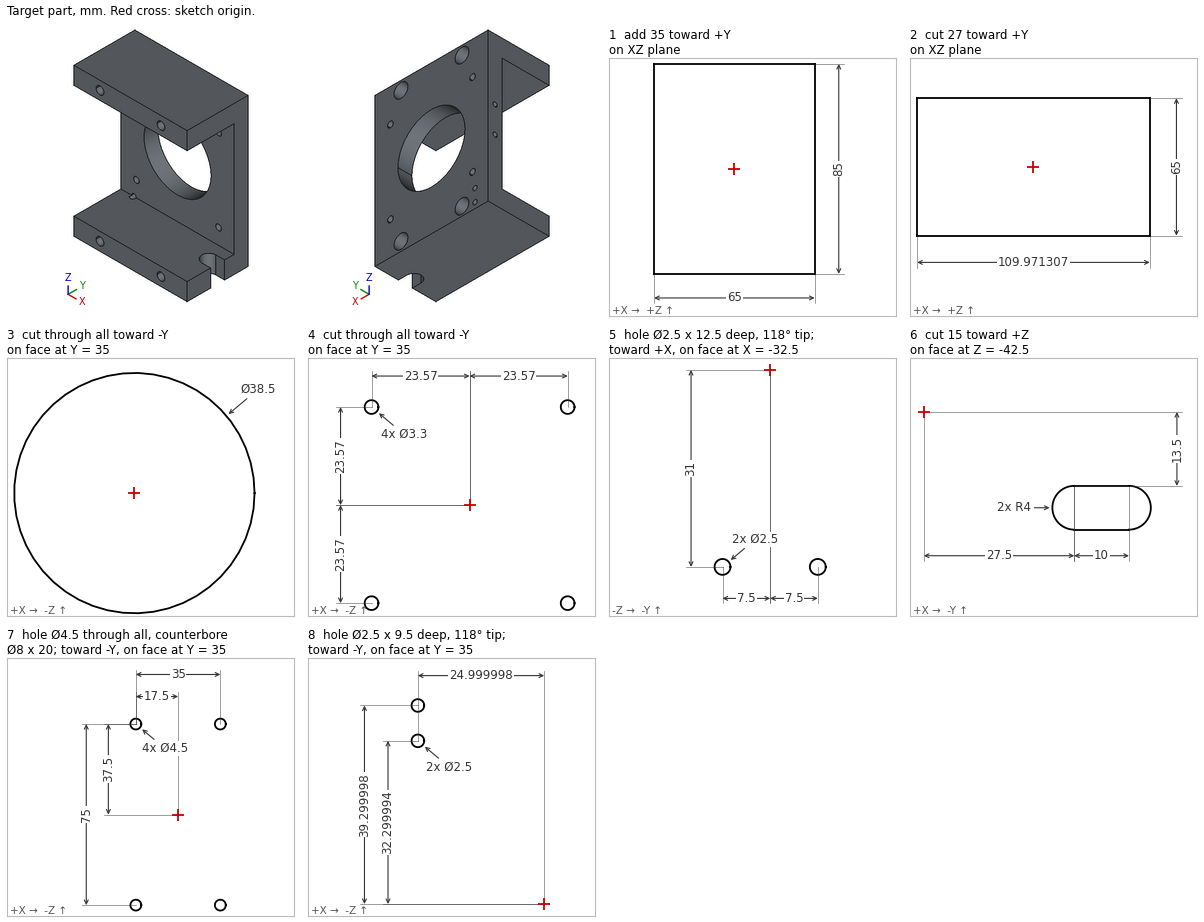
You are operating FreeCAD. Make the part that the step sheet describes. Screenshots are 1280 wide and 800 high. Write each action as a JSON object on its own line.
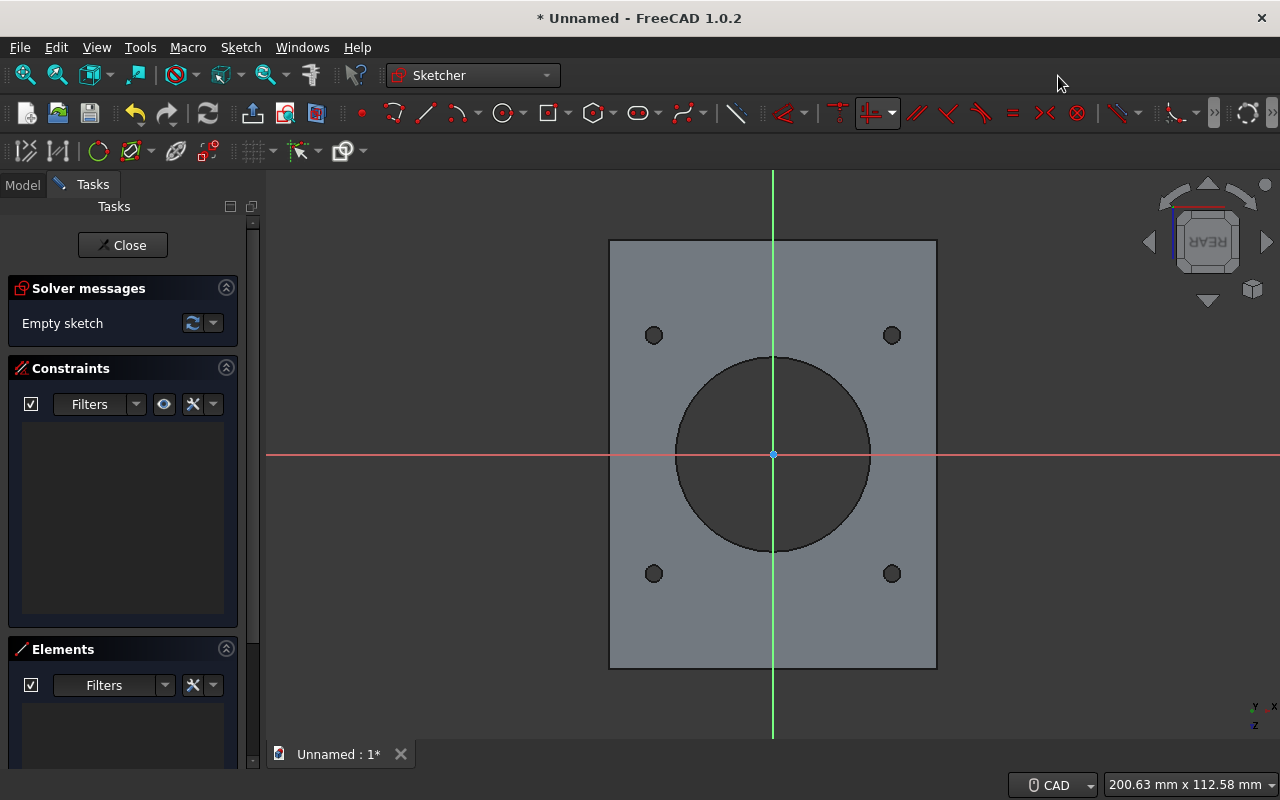
{"action": "left_click", "coordinate": [504, 114]}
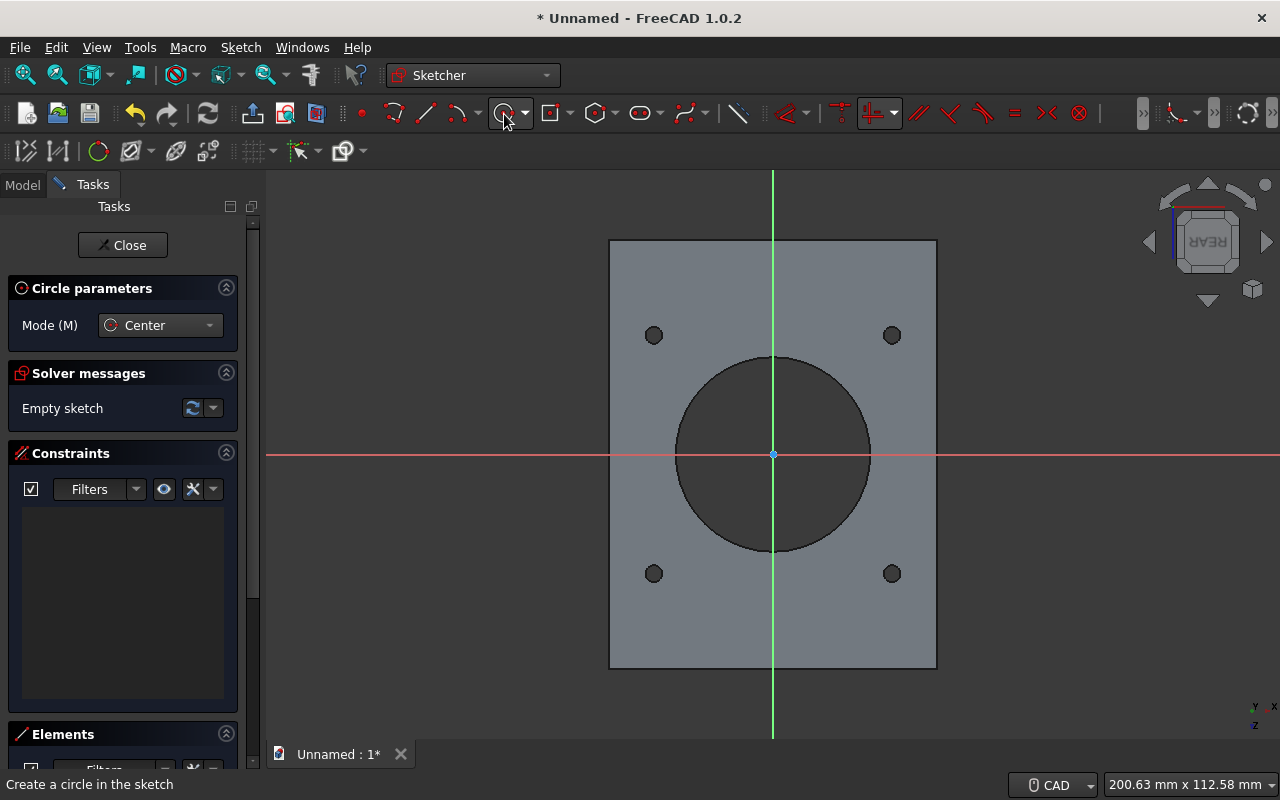
{"action": "scroll", "coordinate": [685, 265], "scroll_direction": "up", "scroll_amount": 4}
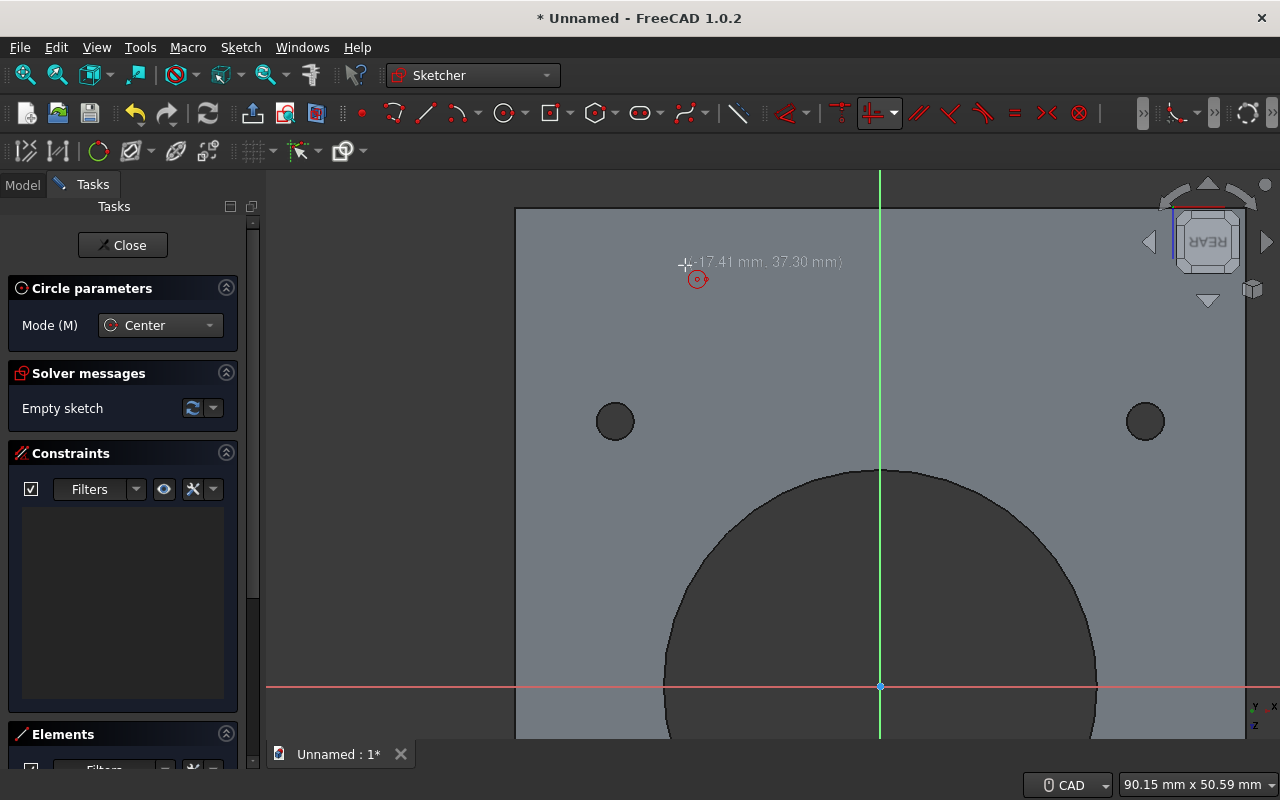
{"action": "left_click", "coordinate": [684, 265]}
{"action": "mouse_move", "coordinate": [701, 247]}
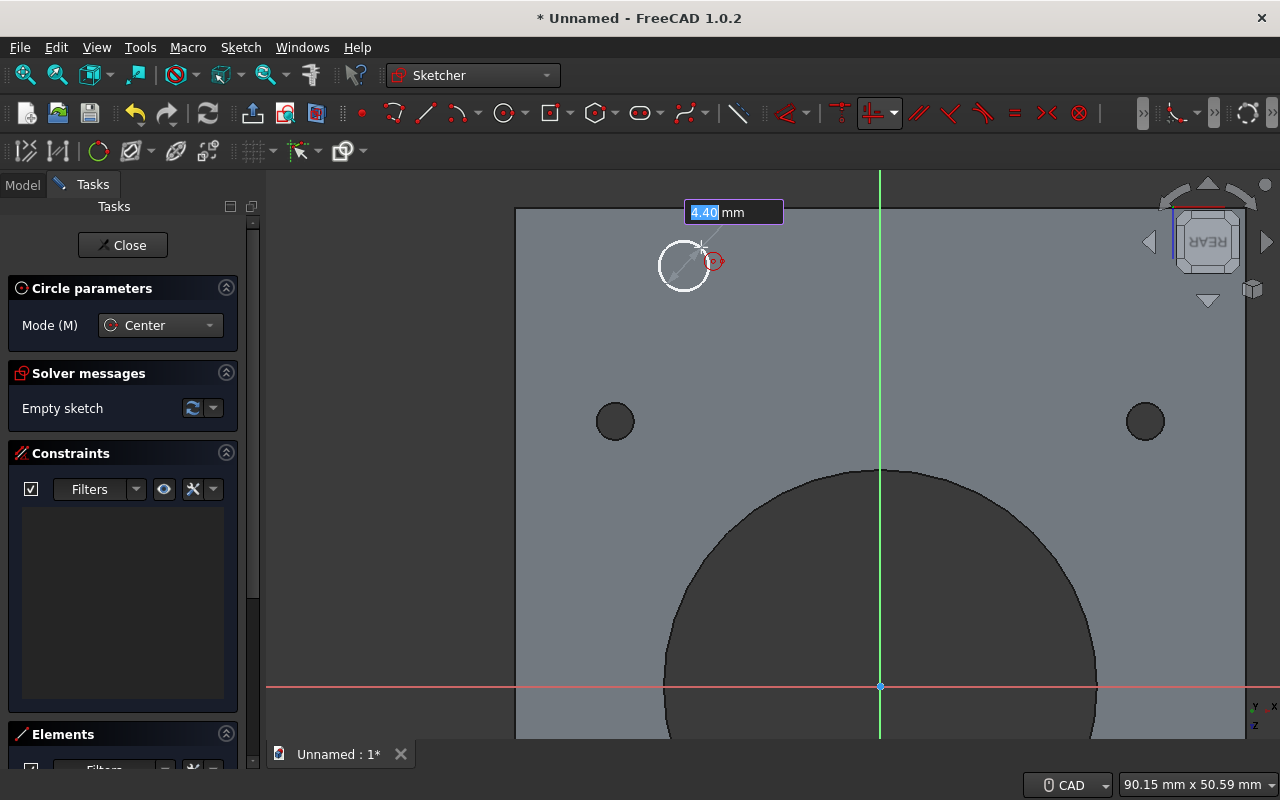
{"action": "type", "text": "4.5"}
{"action": "key", "text": "Return"}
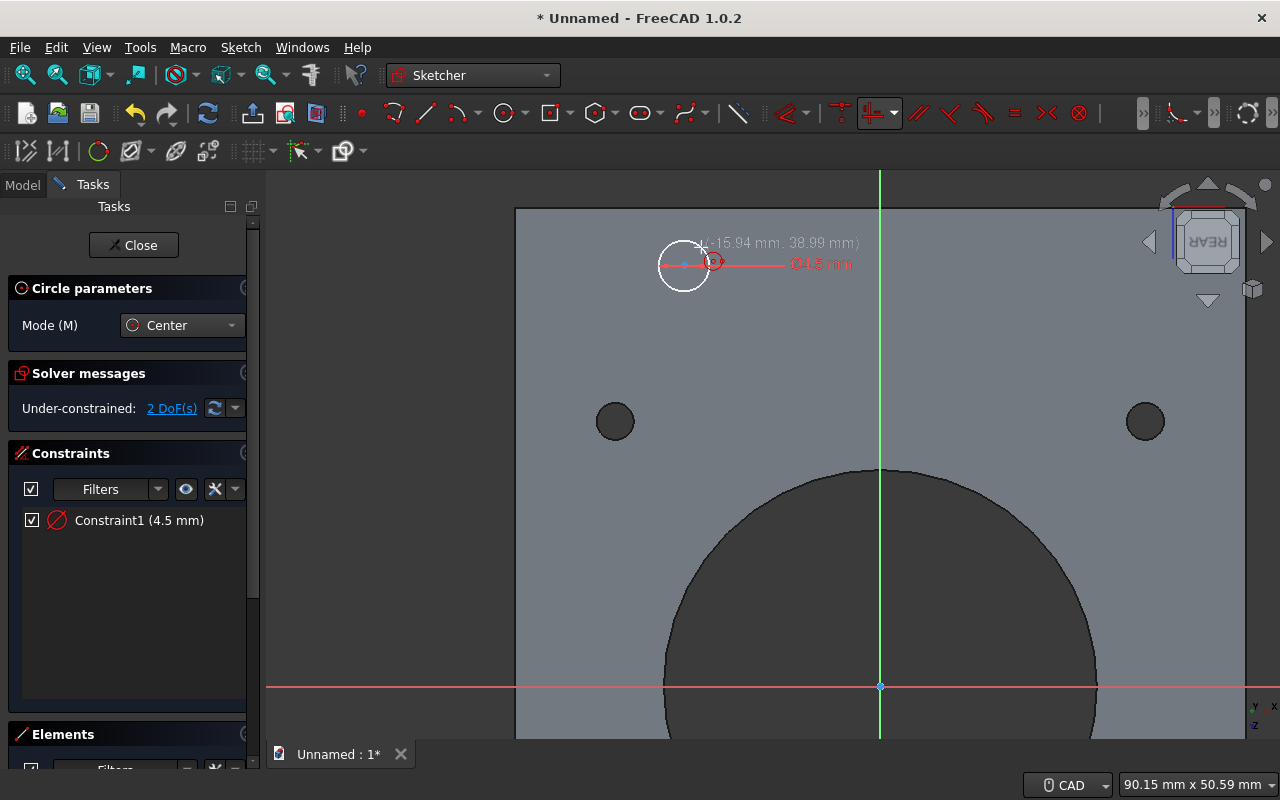
{"action": "left_click", "coordinate": [1077, 265]}
{"action": "mouse_move", "coordinate": [1095, 247]}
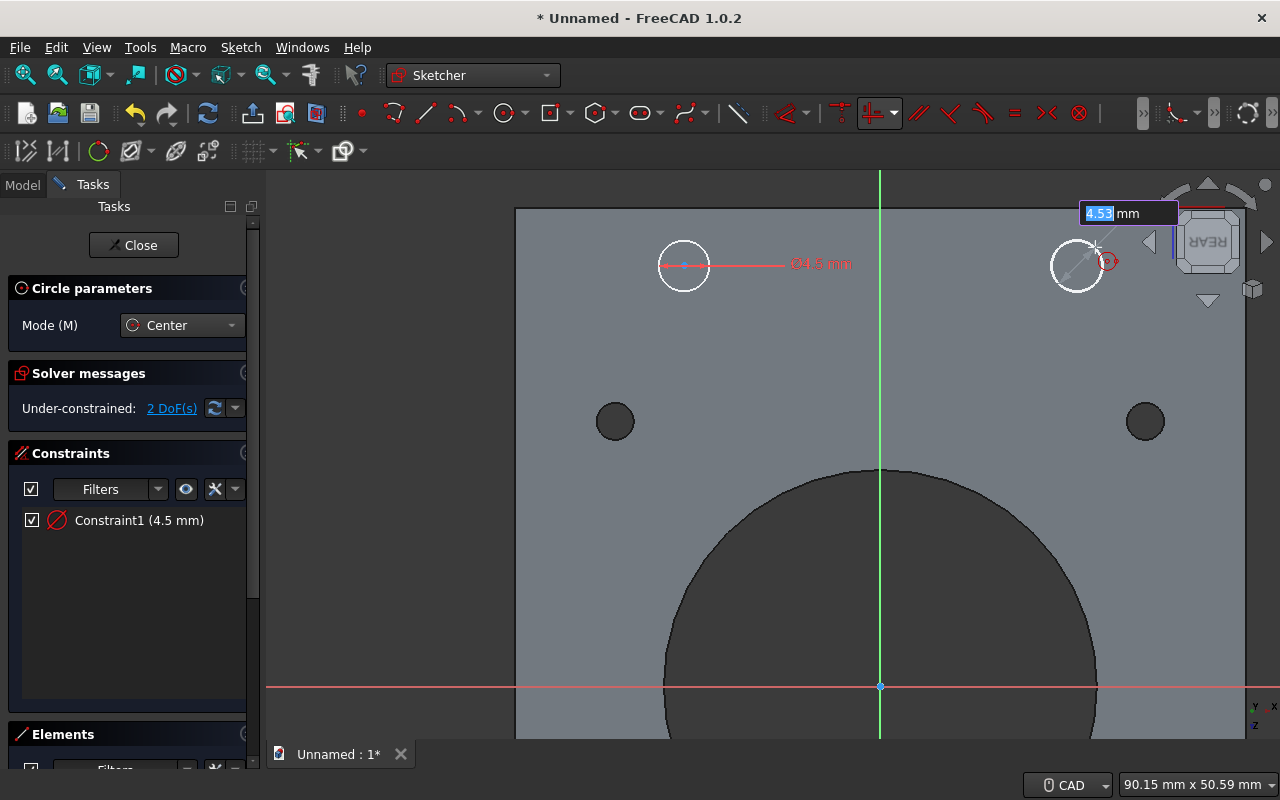
{"action": "type", "text": "4.5"}
{"action": "key", "text": "Return"}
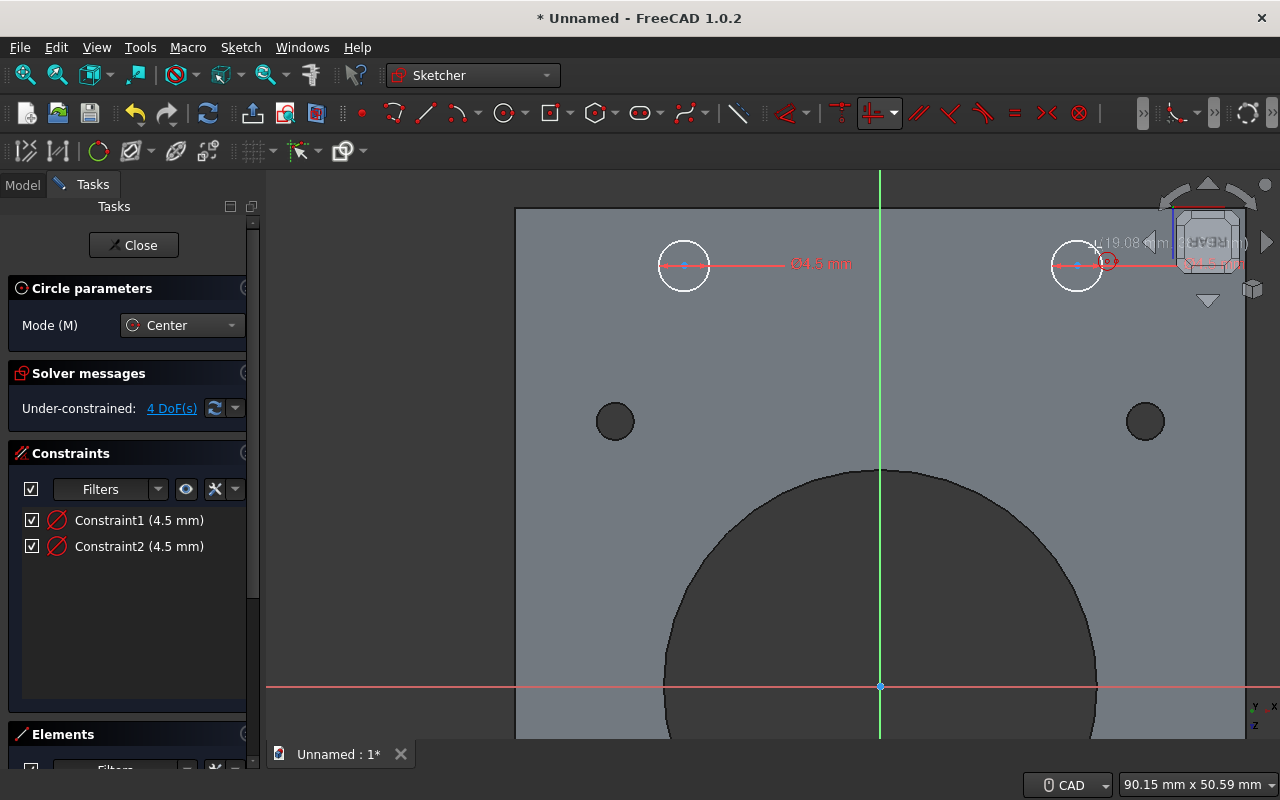
{"action": "scroll", "coordinate": [602, 319], "scroll_direction": "down", "scroll_amount": 5}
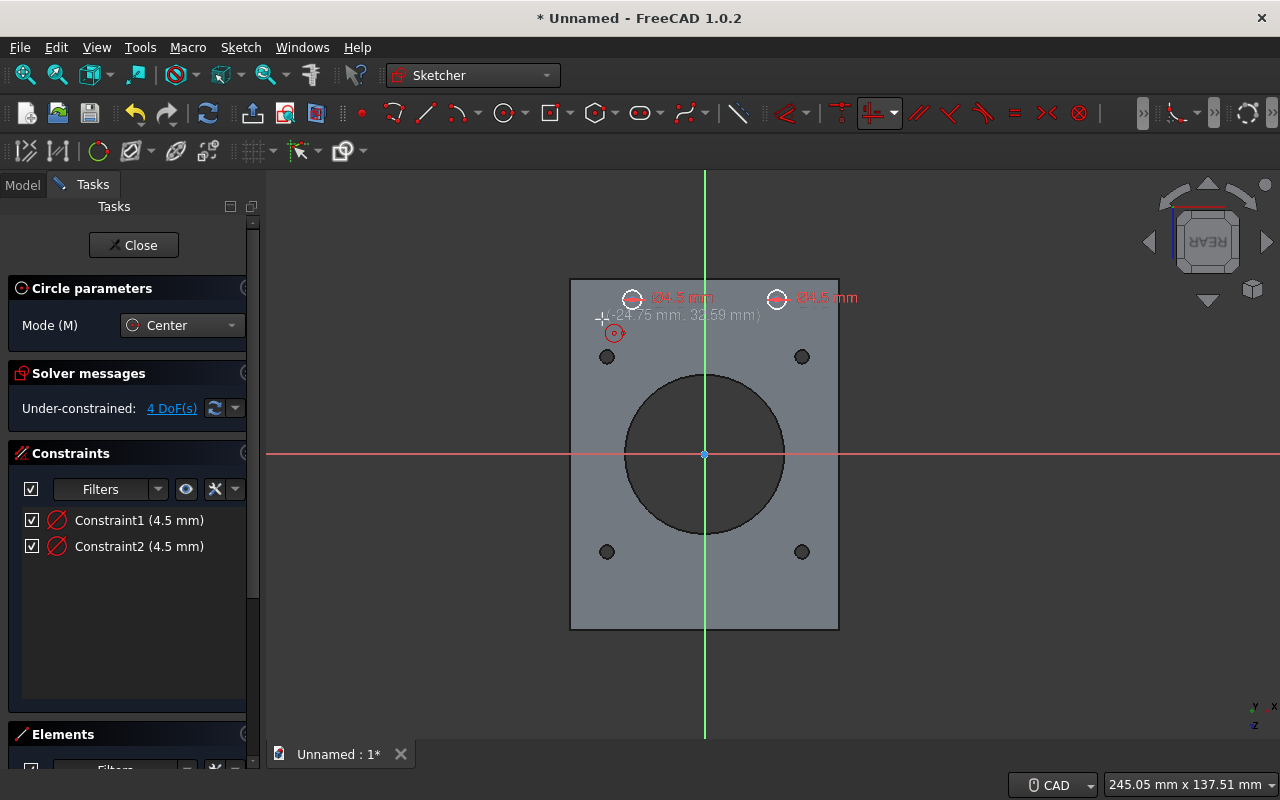
{"action": "scroll", "coordinate": [632, 610], "scroll_direction": "up", "scroll_amount": 5}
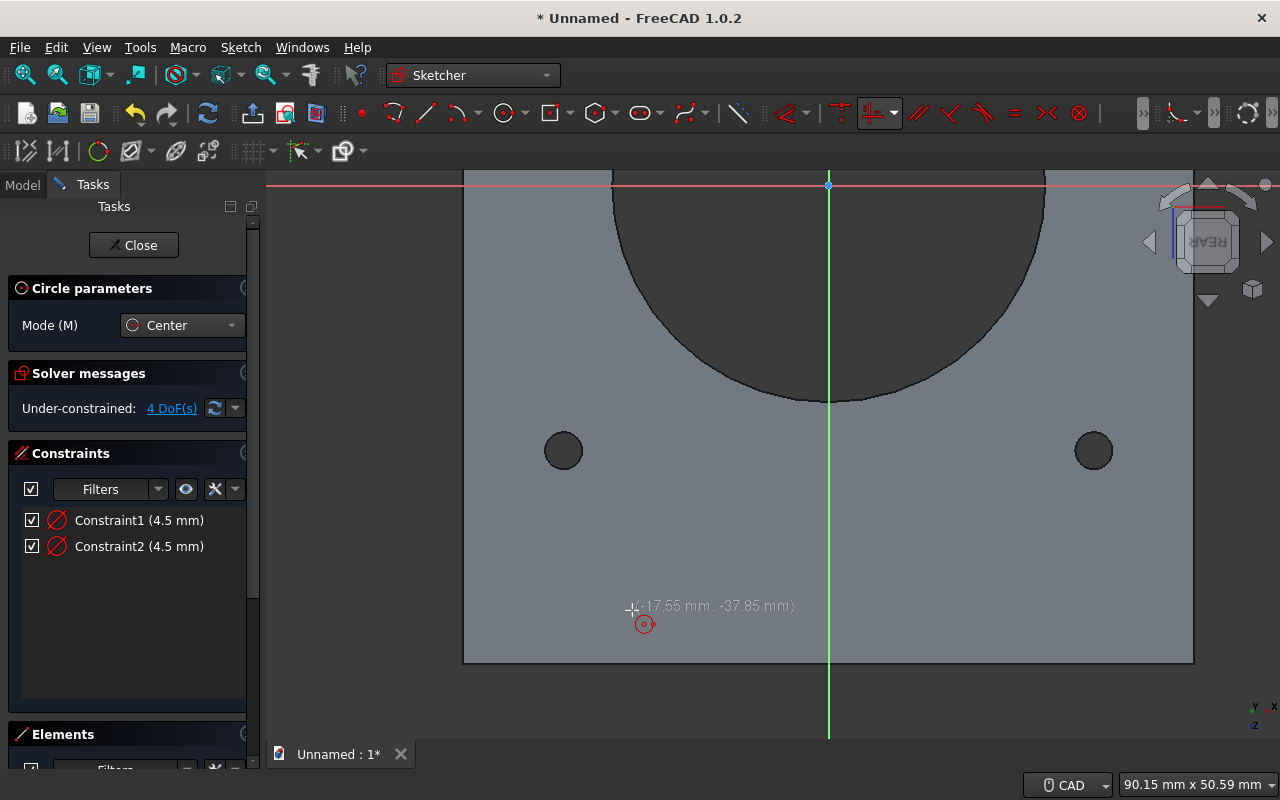
{"action": "left_click", "coordinate": [632, 607]}
{"action": "mouse_move", "coordinate": [650, 590]}